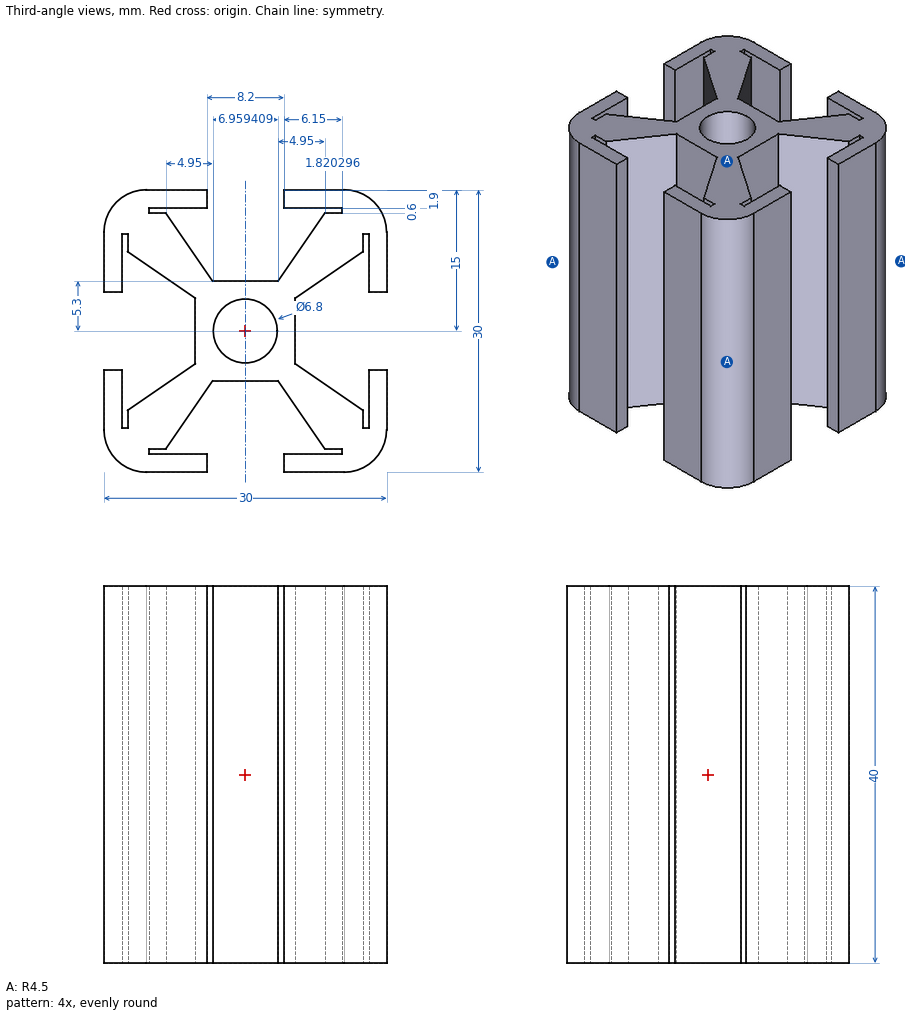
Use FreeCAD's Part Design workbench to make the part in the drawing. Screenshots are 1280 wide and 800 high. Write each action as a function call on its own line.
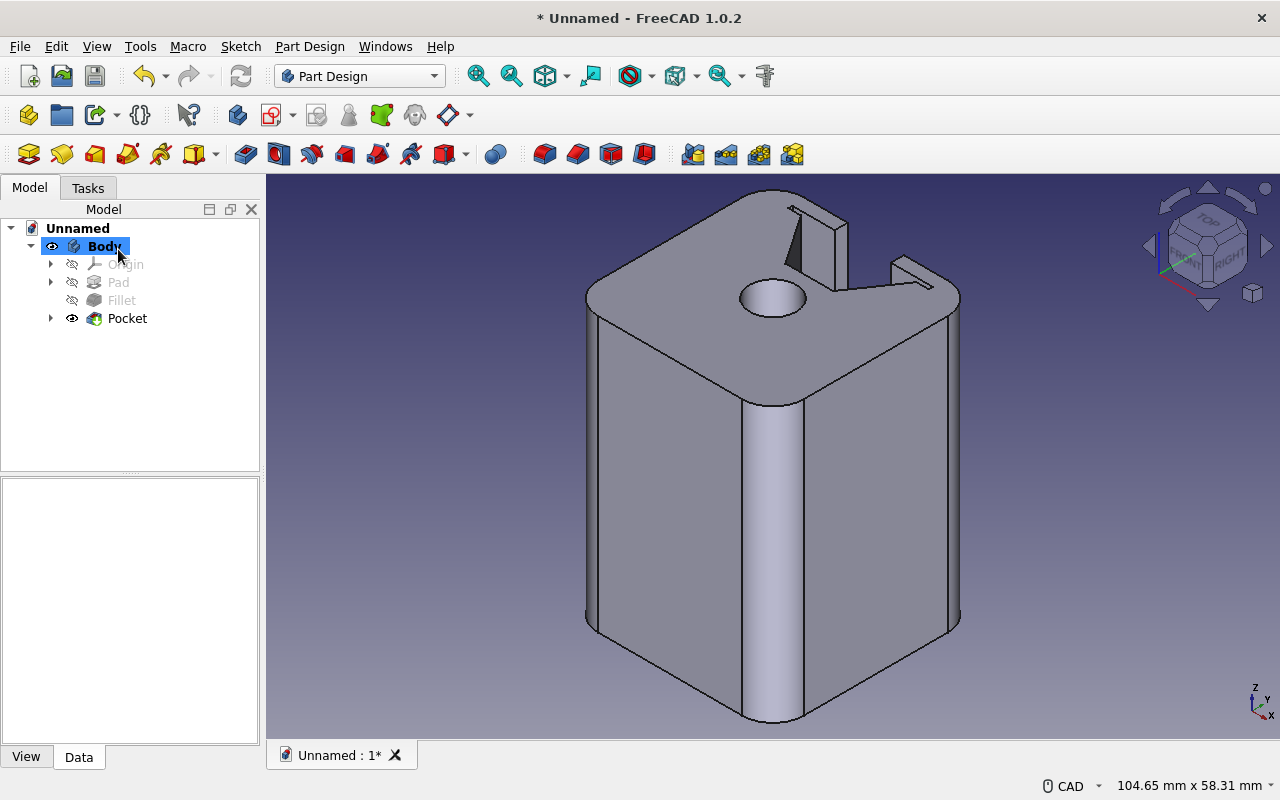
click(117, 318)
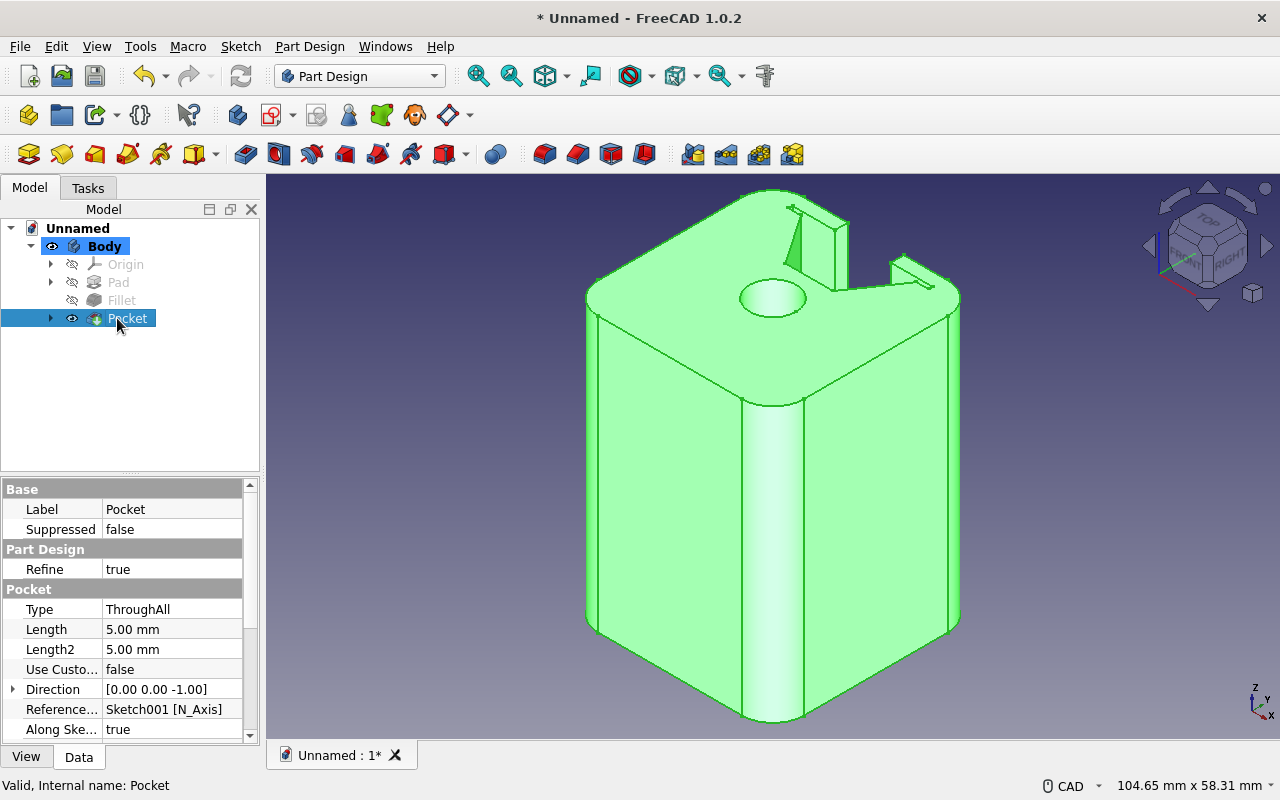
click(759, 154)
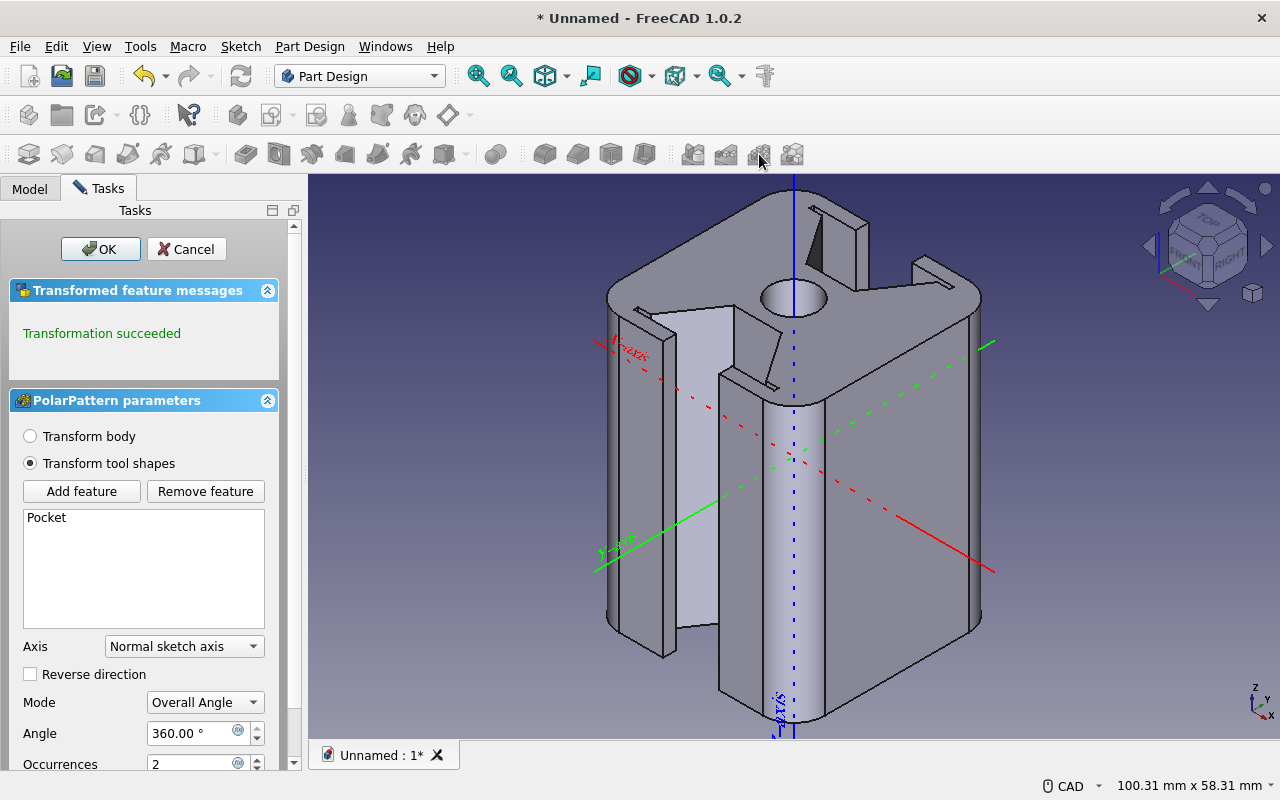
click(185, 646)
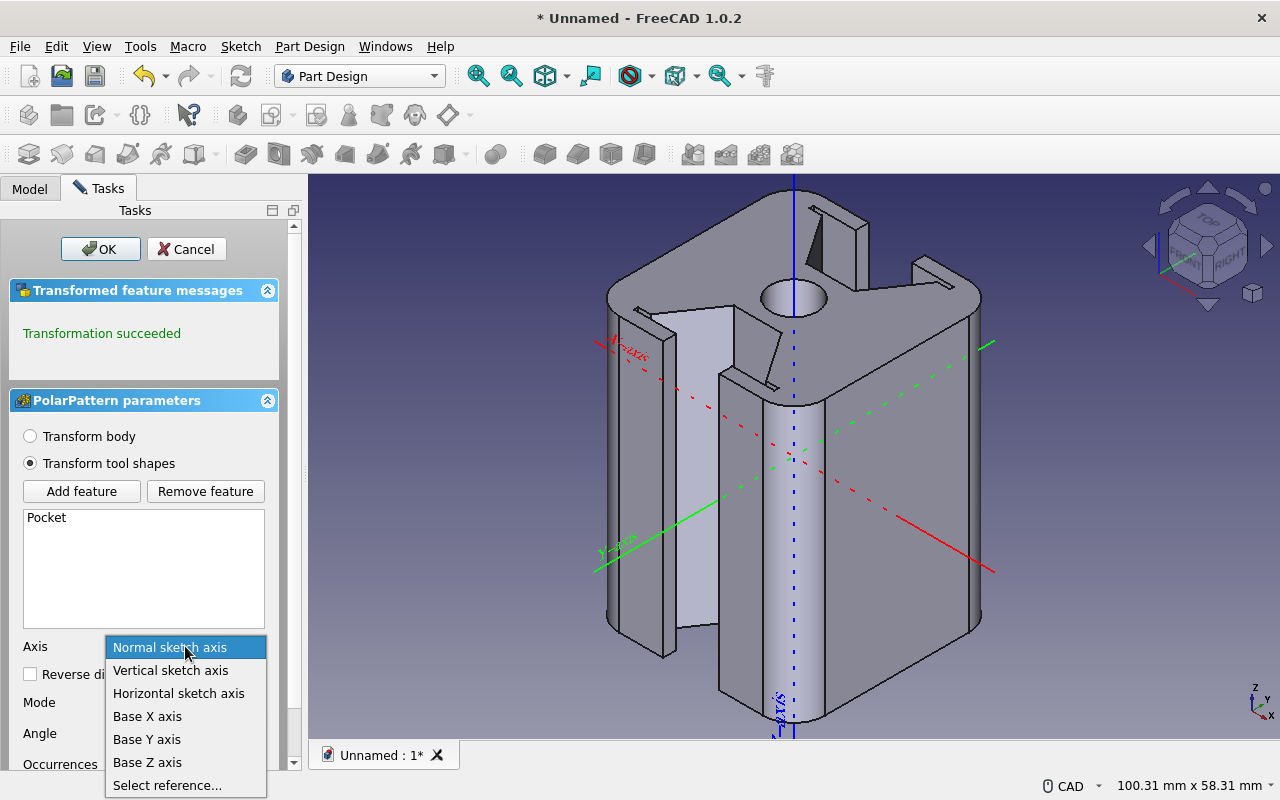
click(184, 762)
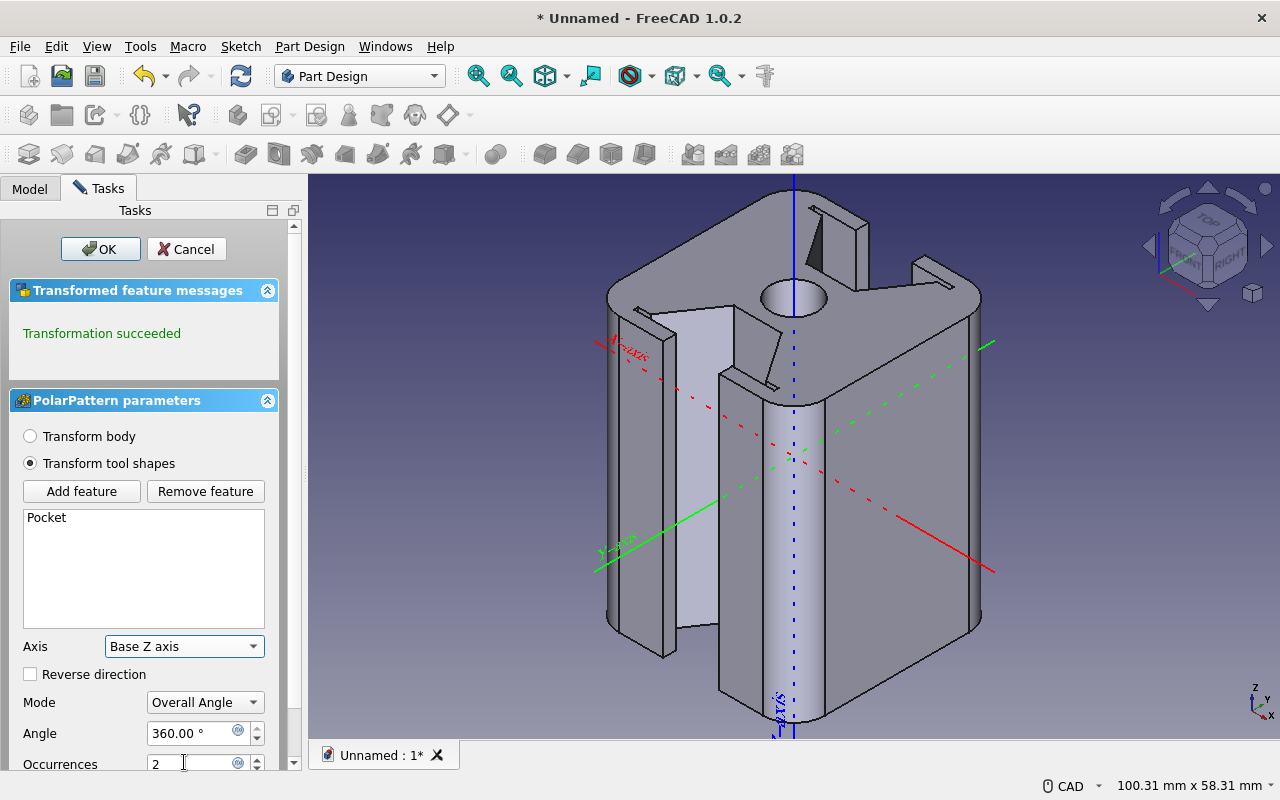
scroll(294, 495, down, 2)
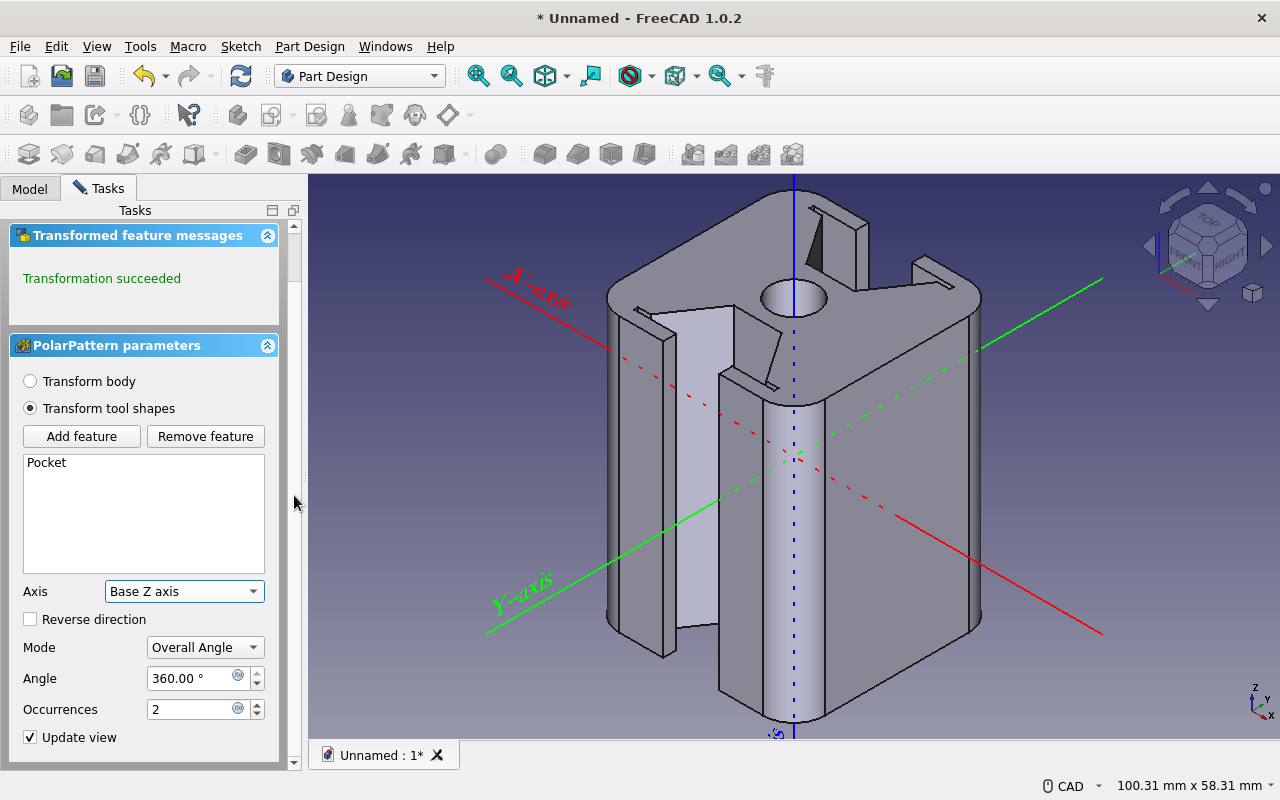
triple_click(199, 710)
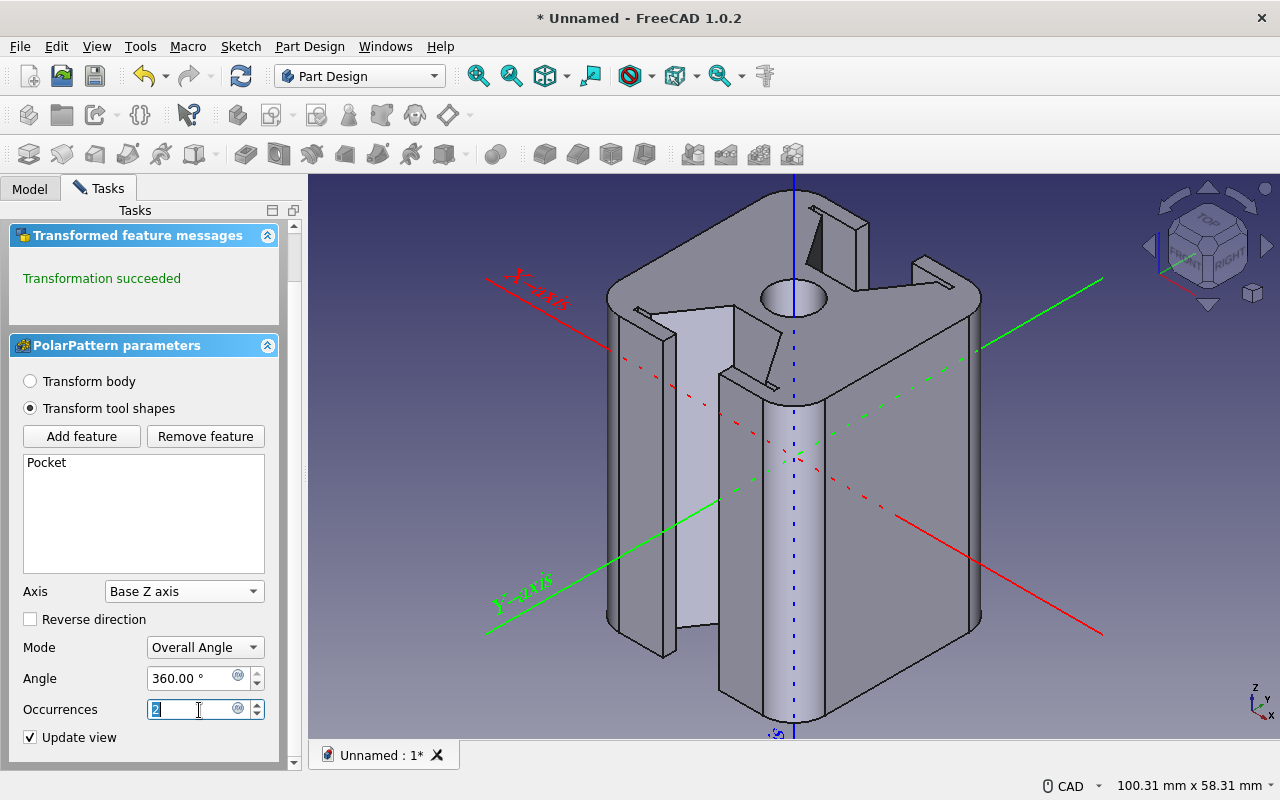
text(4)
key(Tab)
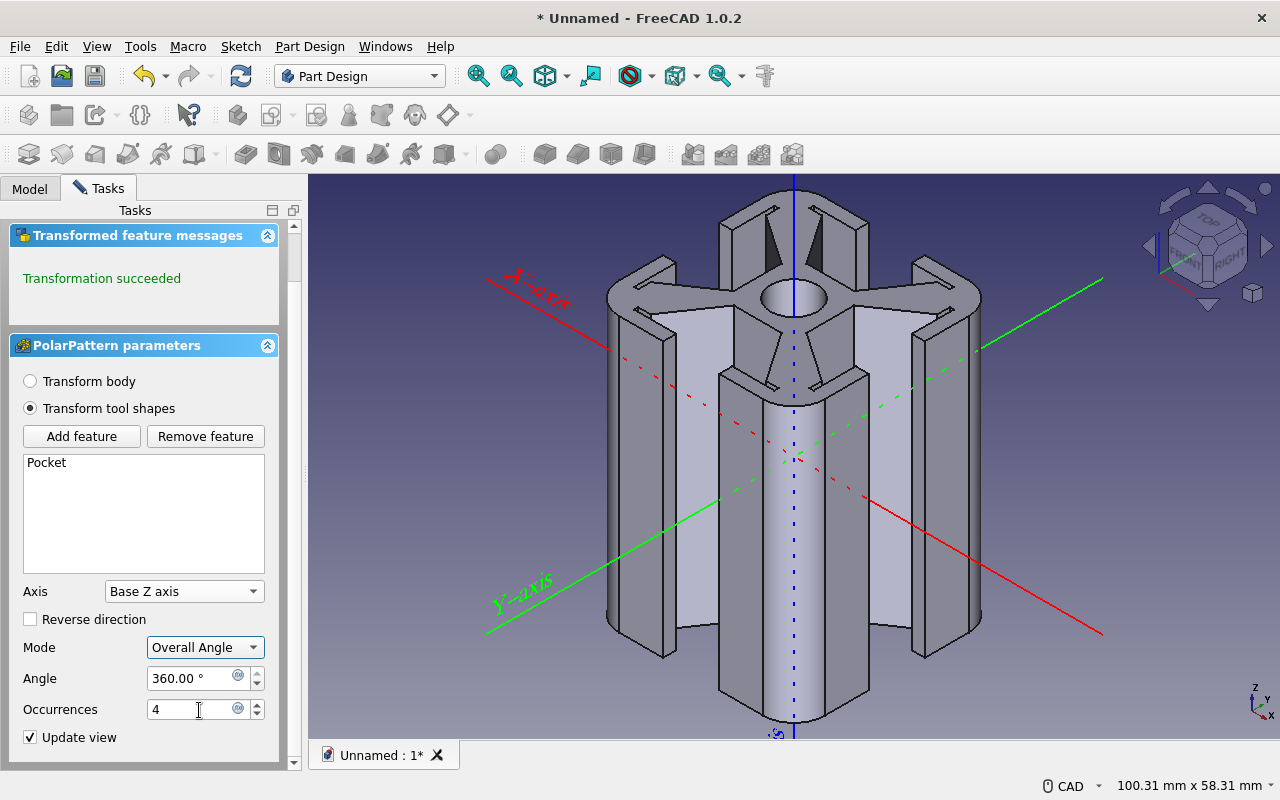
scroll(294, 495, up, 2)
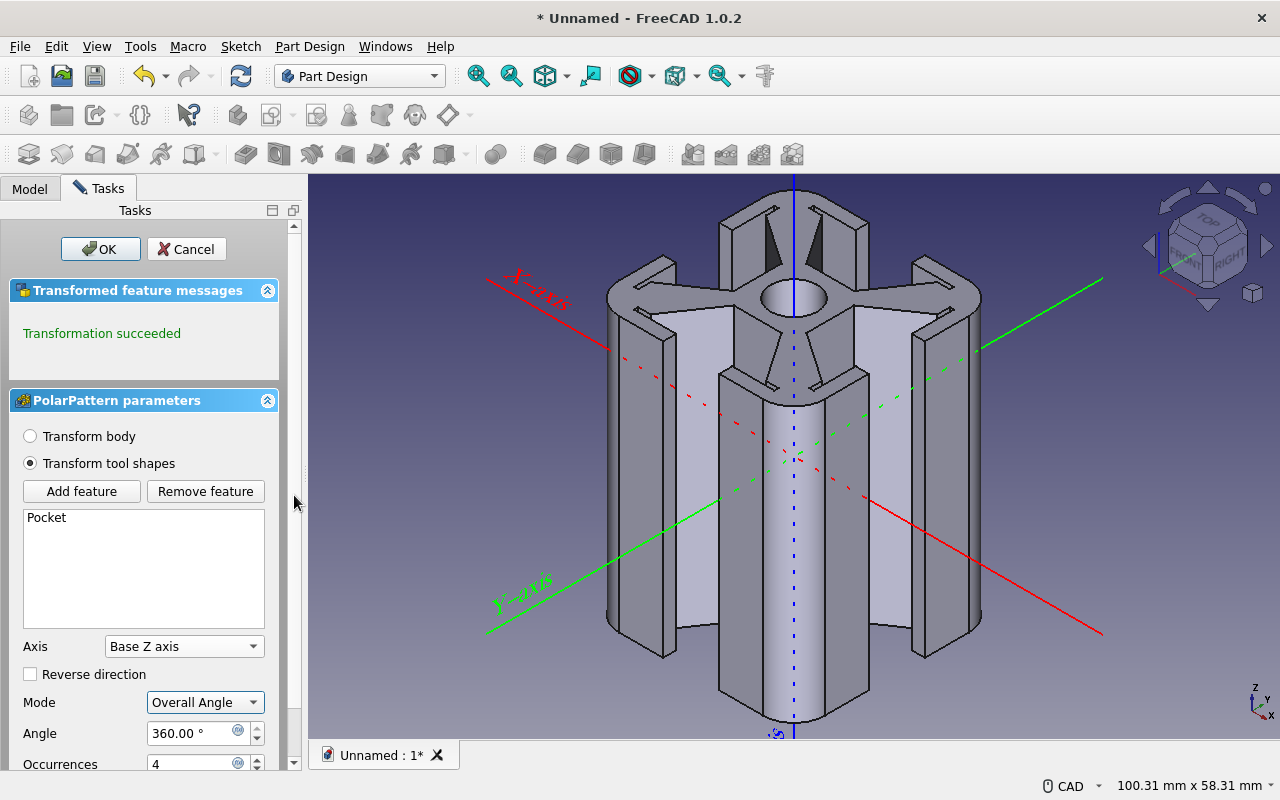
click(101, 249)